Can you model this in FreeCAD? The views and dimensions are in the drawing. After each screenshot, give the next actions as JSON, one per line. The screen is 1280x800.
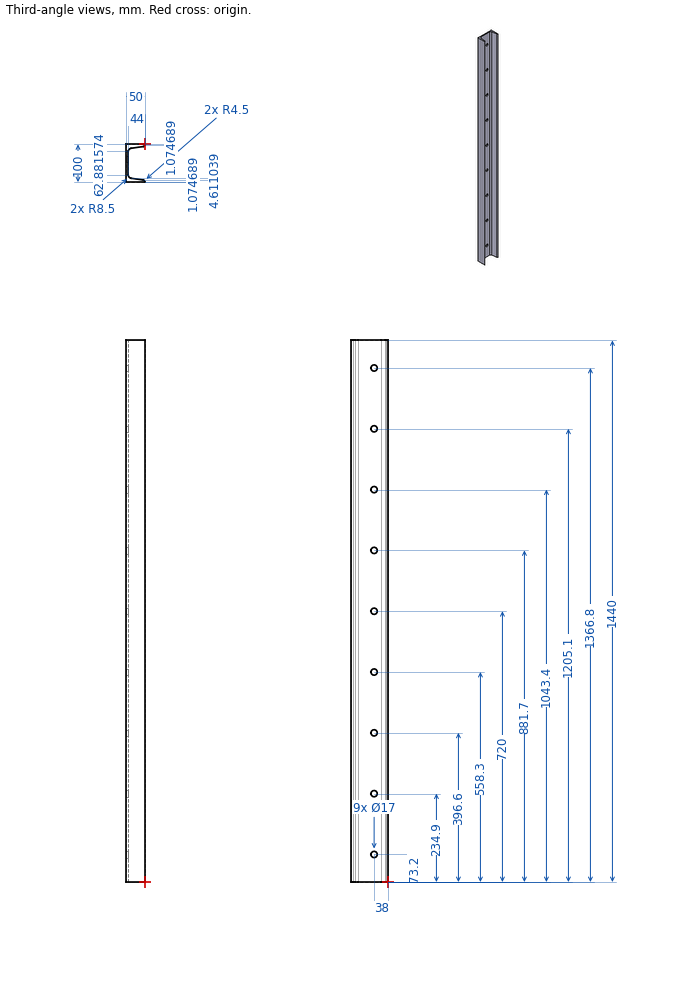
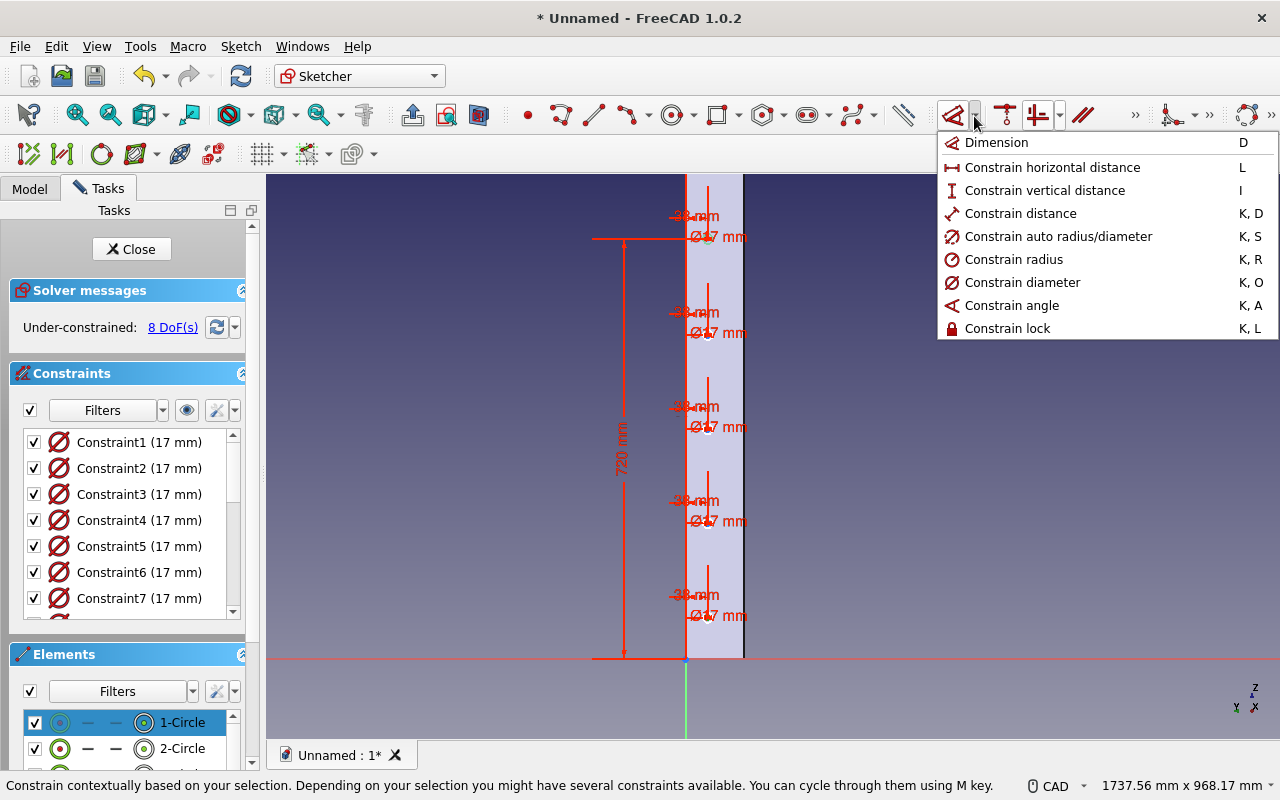
{"action": "left_click", "coordinate": [1108, 190]}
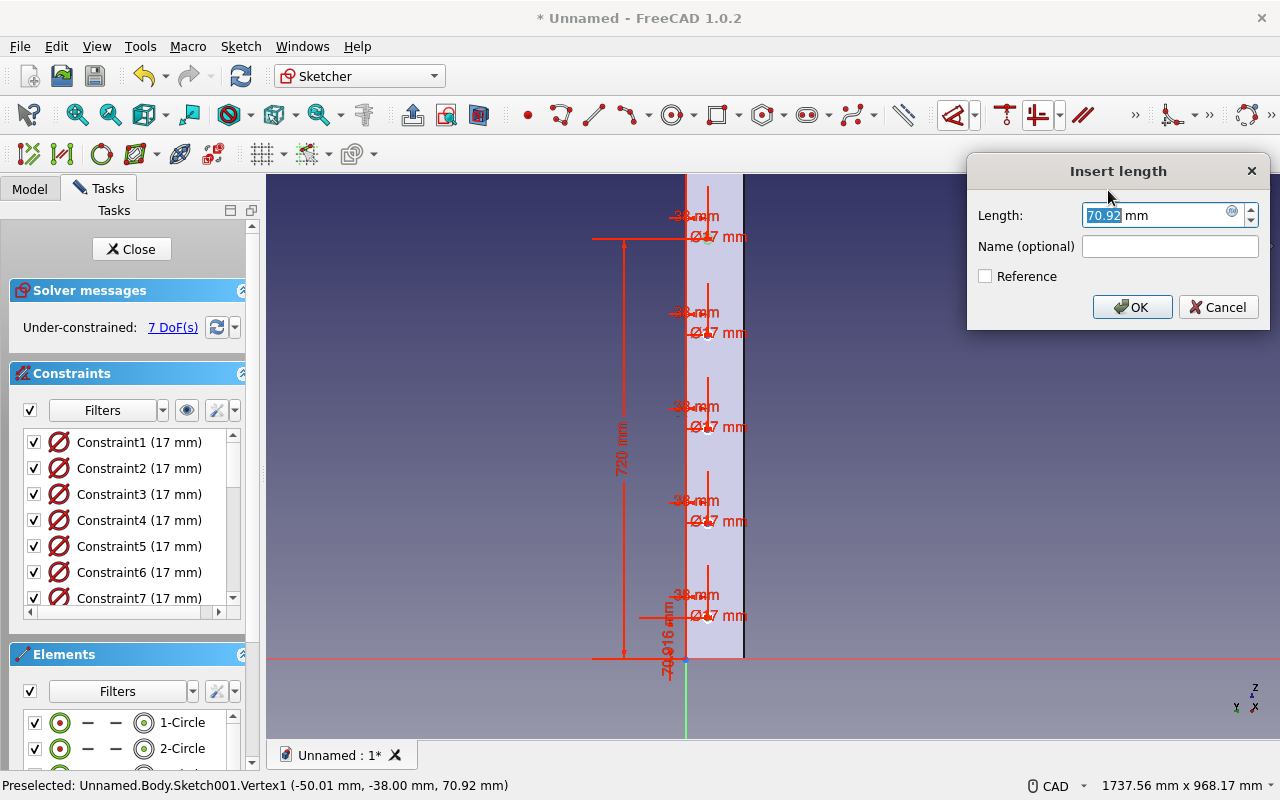
{"action": "type", "text": "73.2"}
{"action": "key", "text": "Return"}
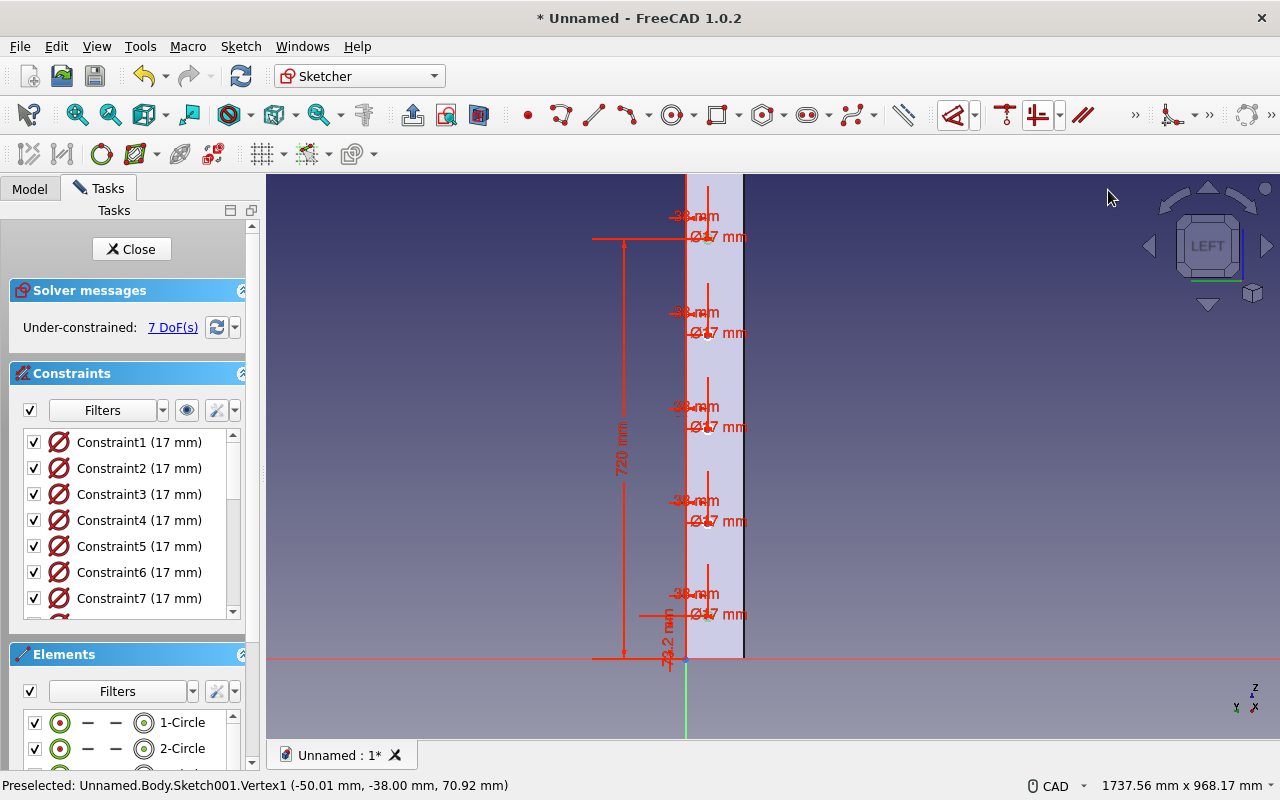
{"action": "left_click", "coordinate": [708, 523]}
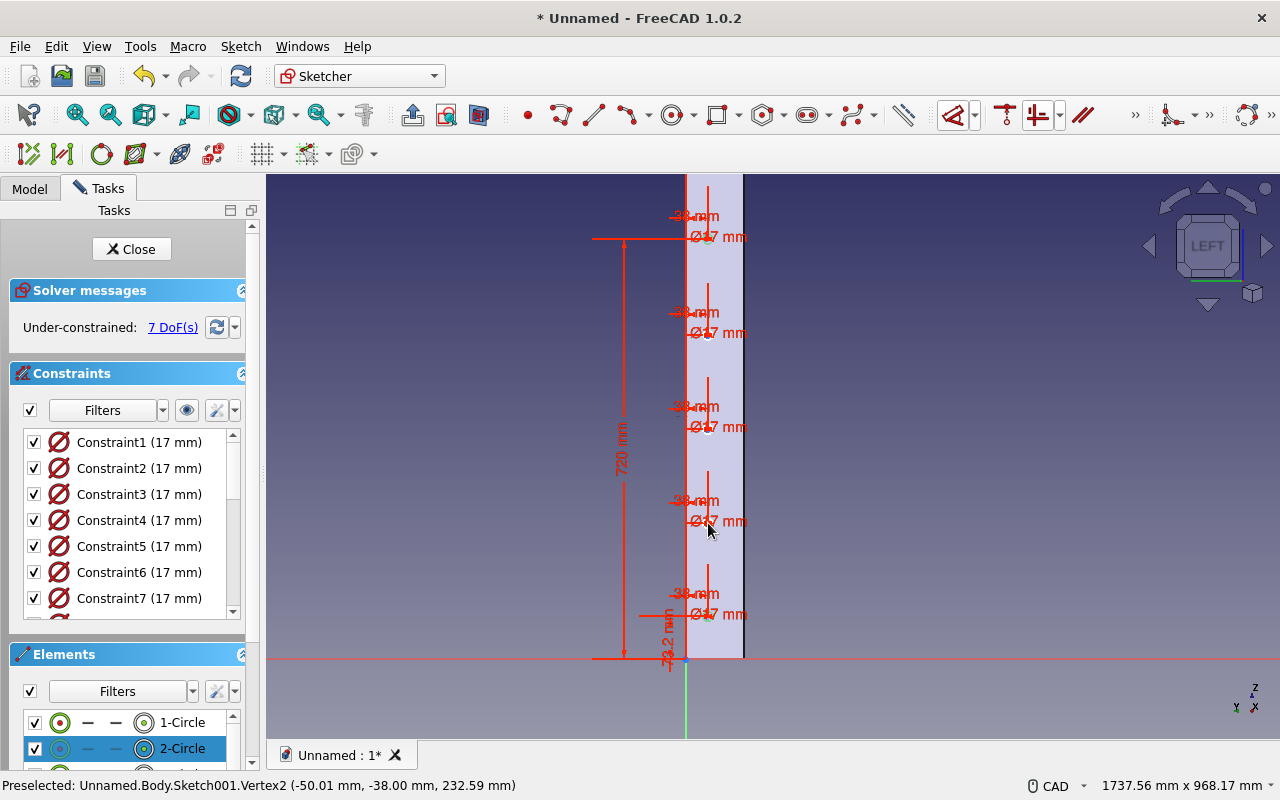
{"action": "left_click", "coordinate": [974, 116]}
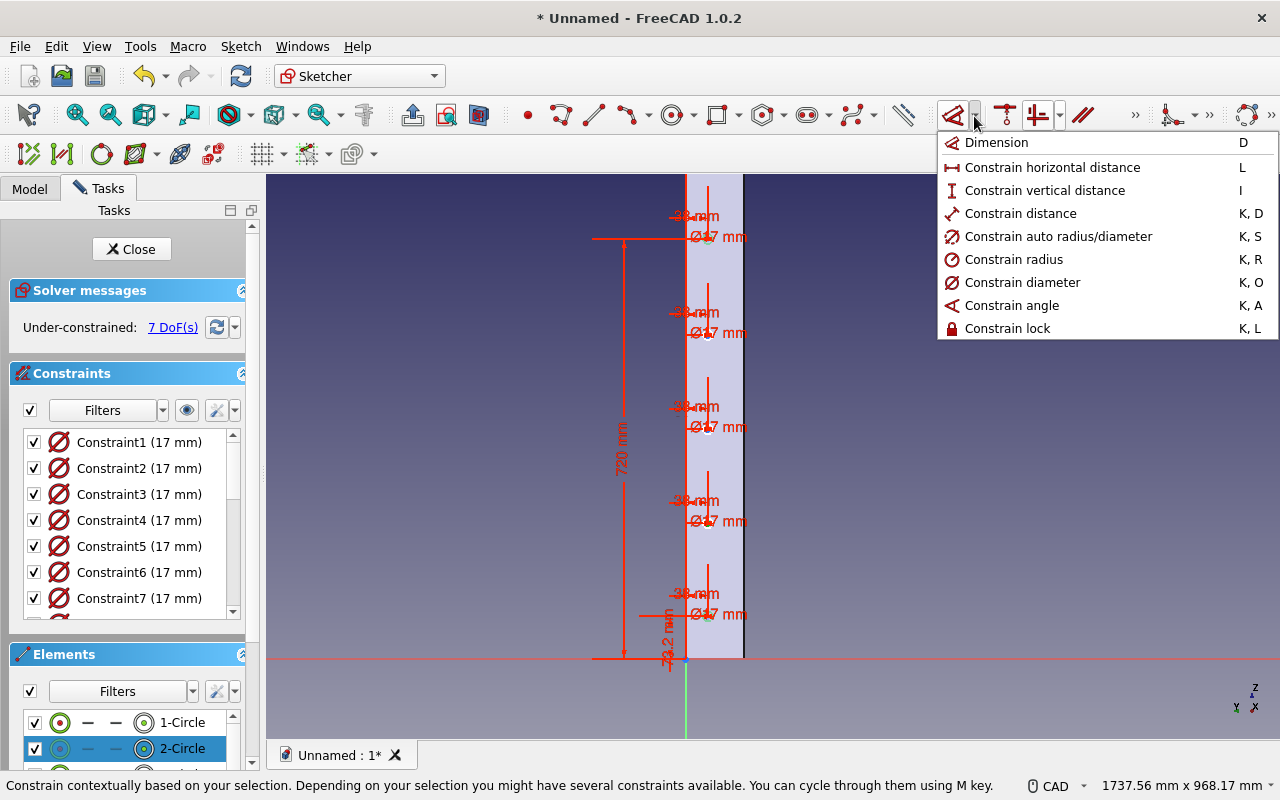
{"action": "left_click", "coordinate": [1108, 190]}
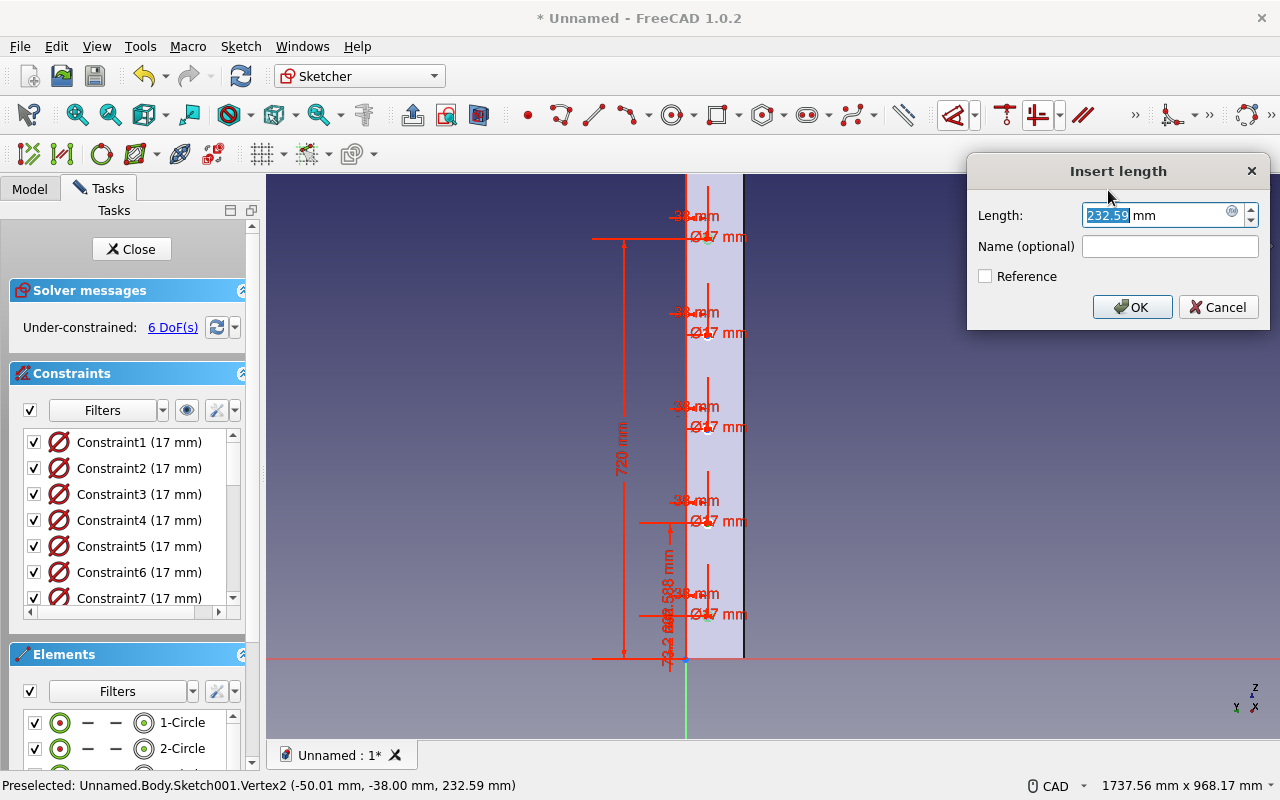
{"action": "type", "text": "234.9"}
{"action": "key", "text": "Return"}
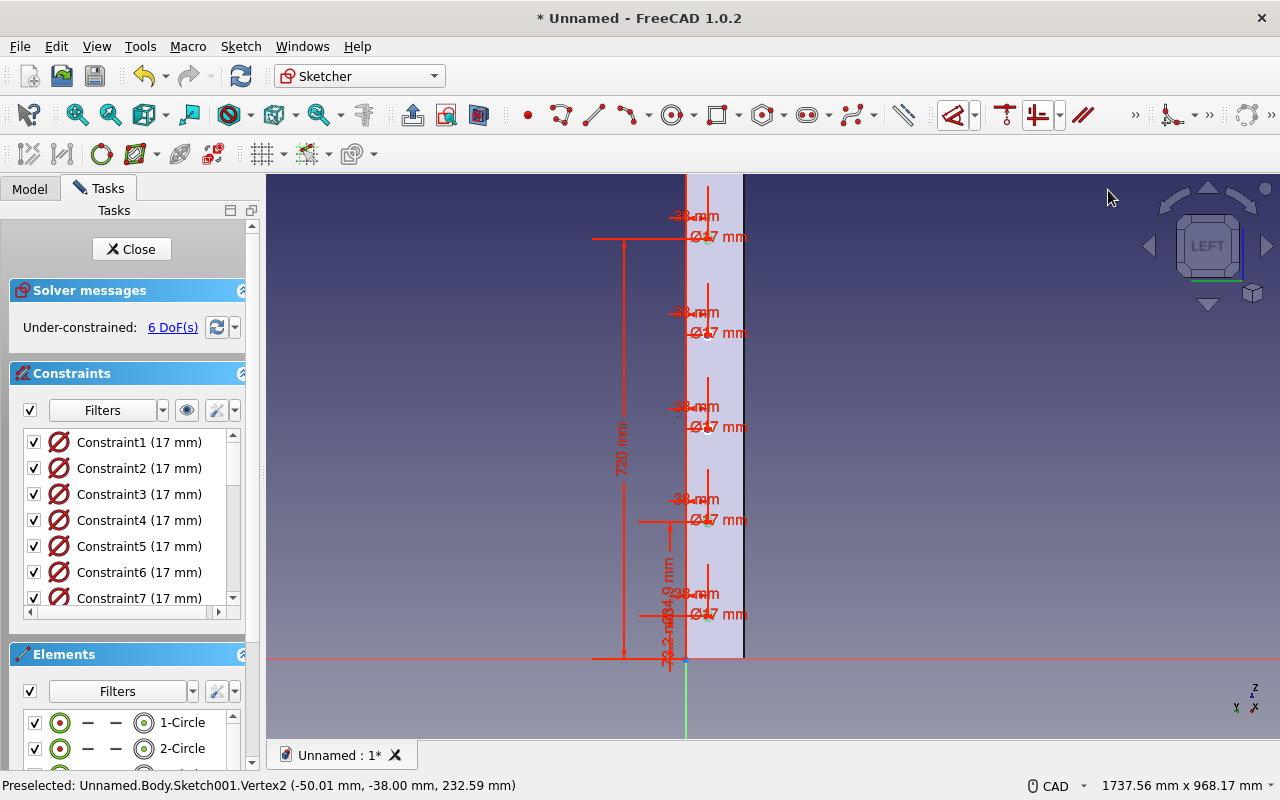
{"action": "left_click", "coordinate": [708, 429]}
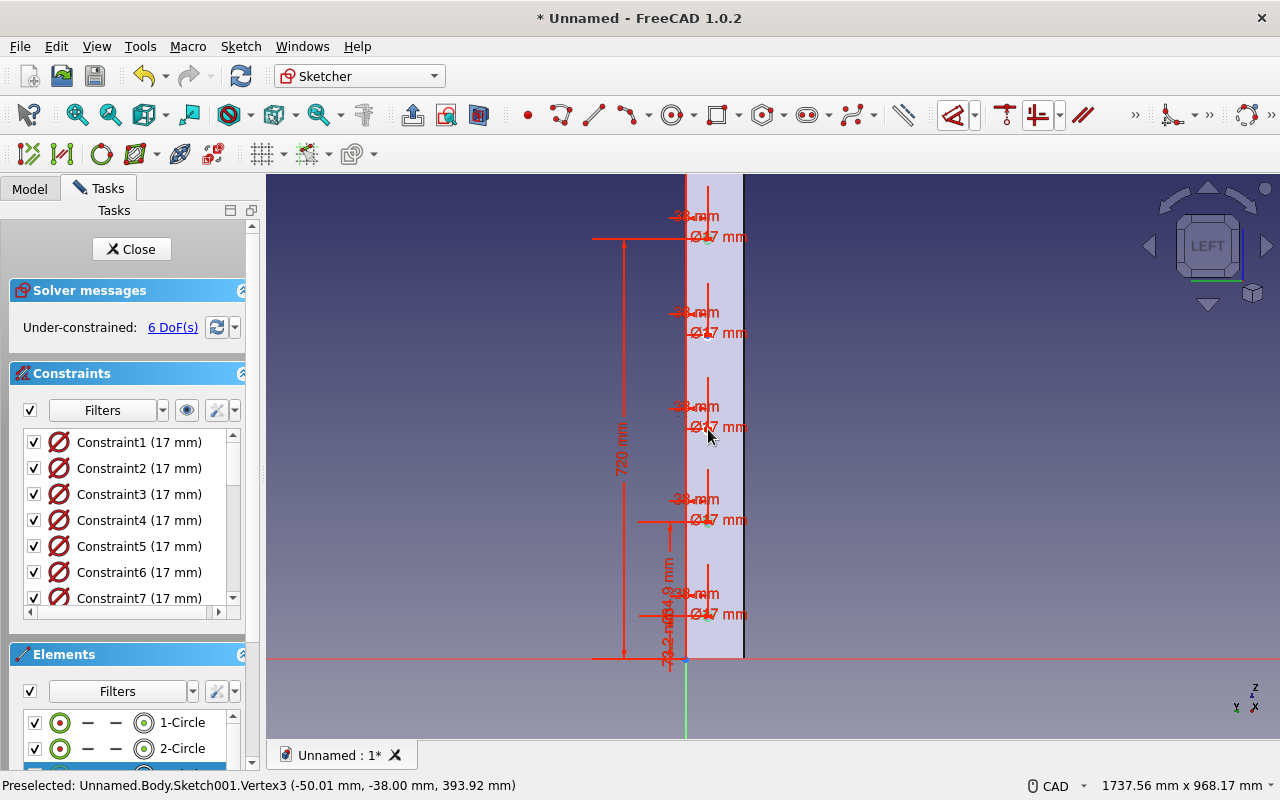
{"action": "key", "text": "i"}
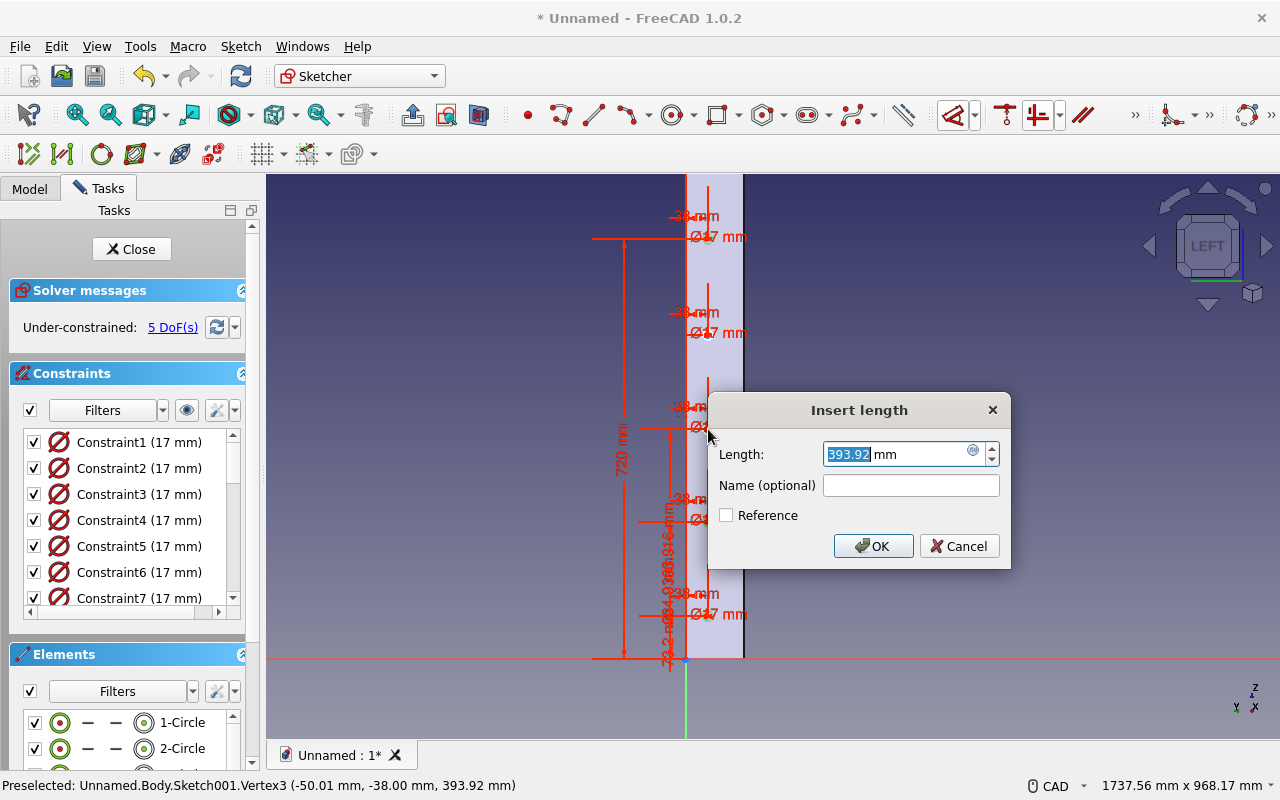
{"action": "type", "text": "396.6"}
{"action": "key", "text": "Return"}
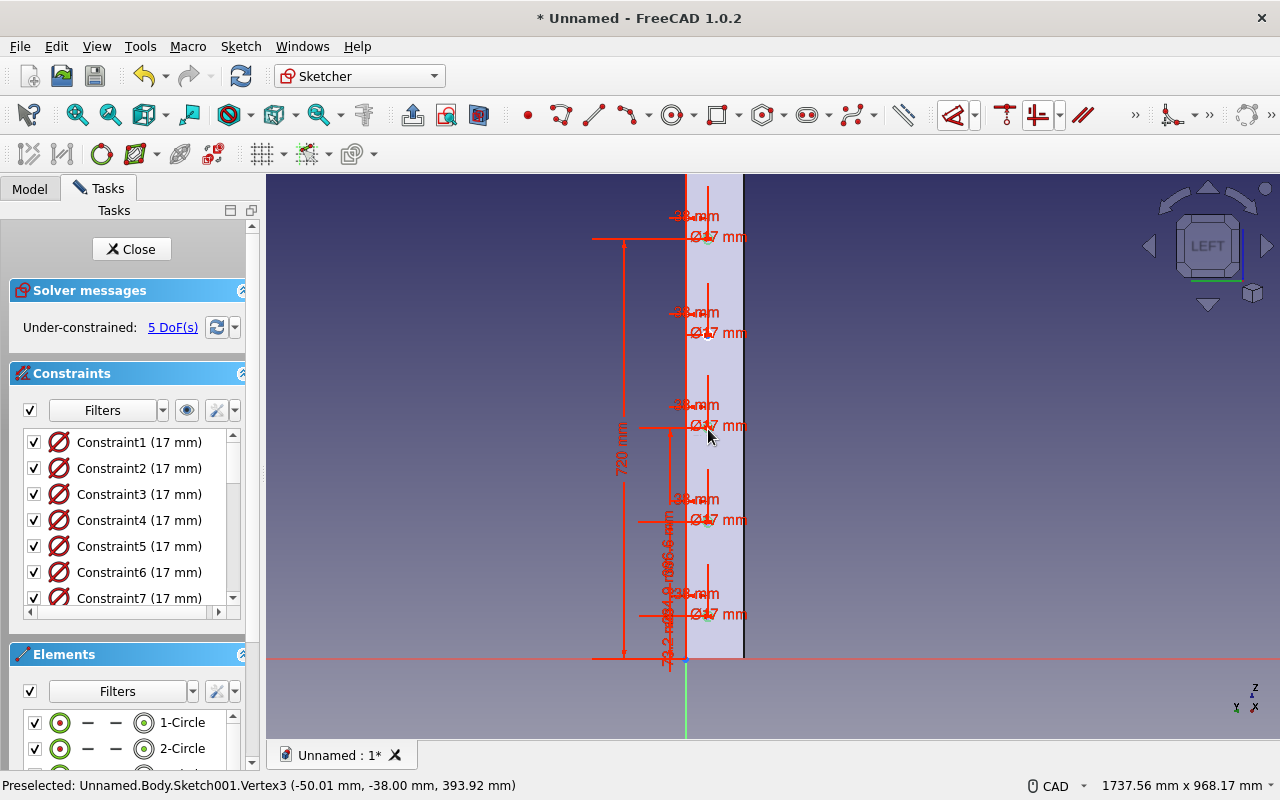
{"action": "left_click", "coordinate": [708, 335]}